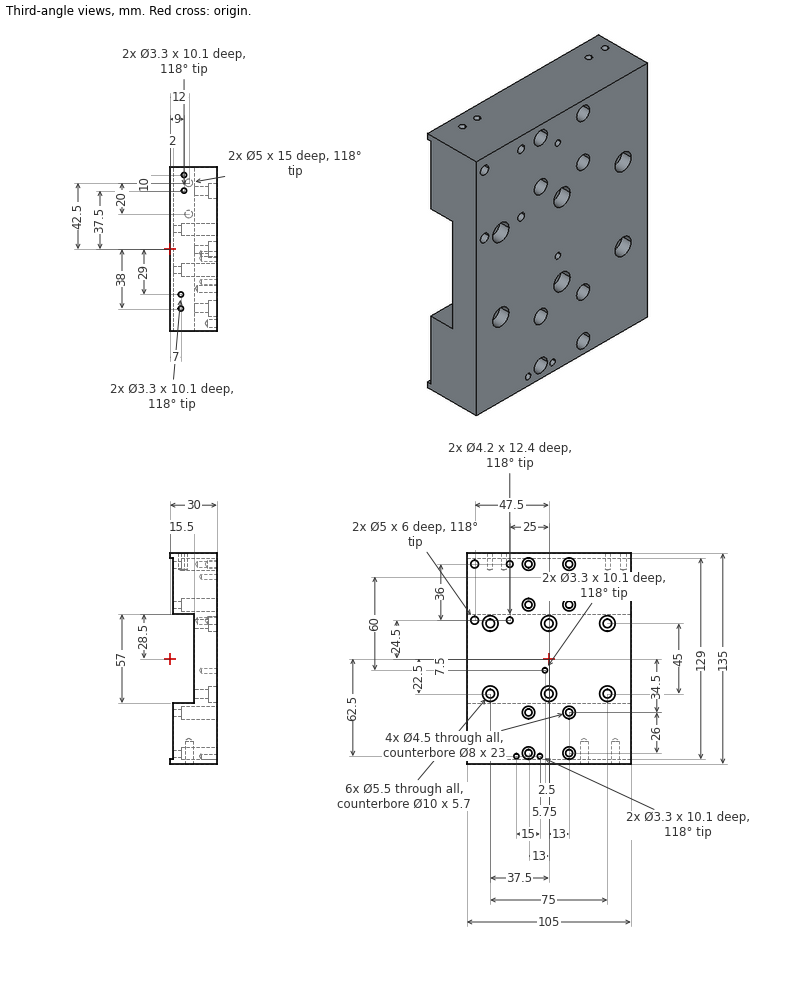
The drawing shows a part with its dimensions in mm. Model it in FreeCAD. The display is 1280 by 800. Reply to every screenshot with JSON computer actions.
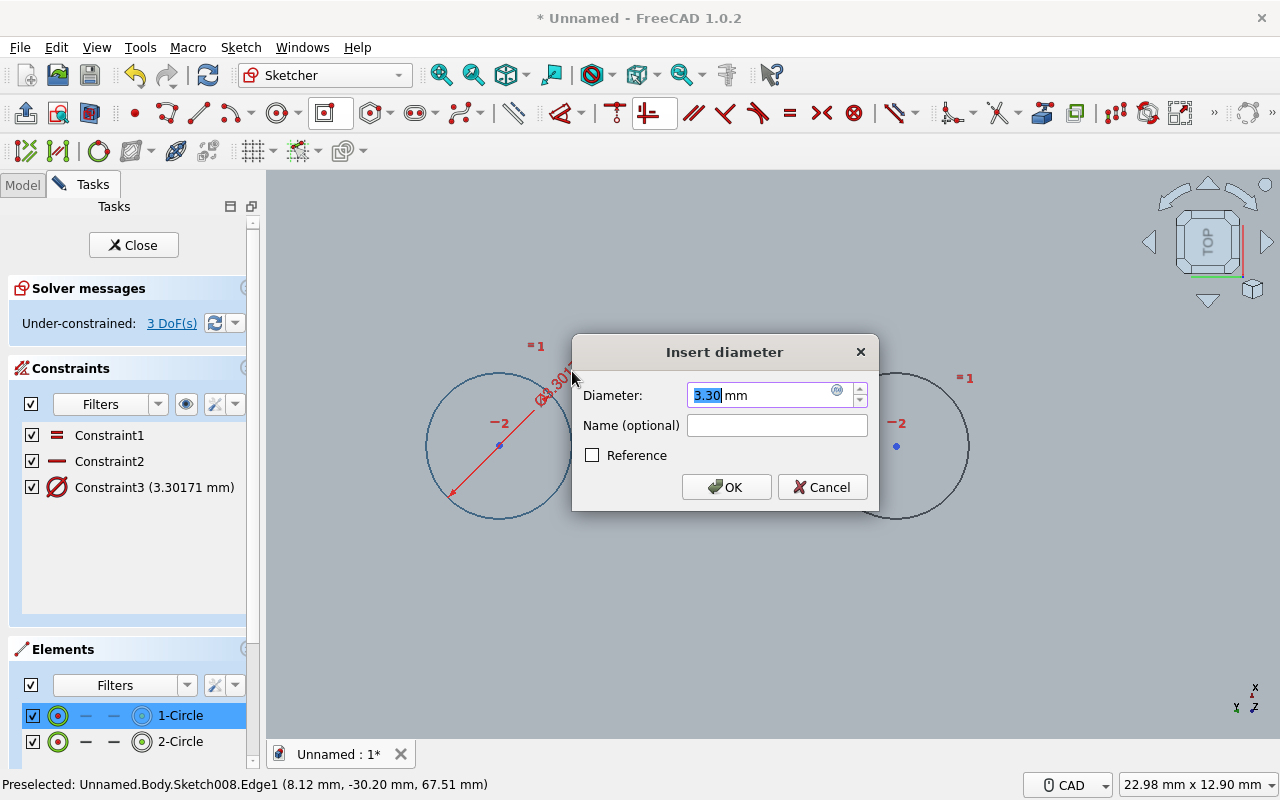
{"action": "type", "text": "3.3"}
{"action": "key", "text": "Return"}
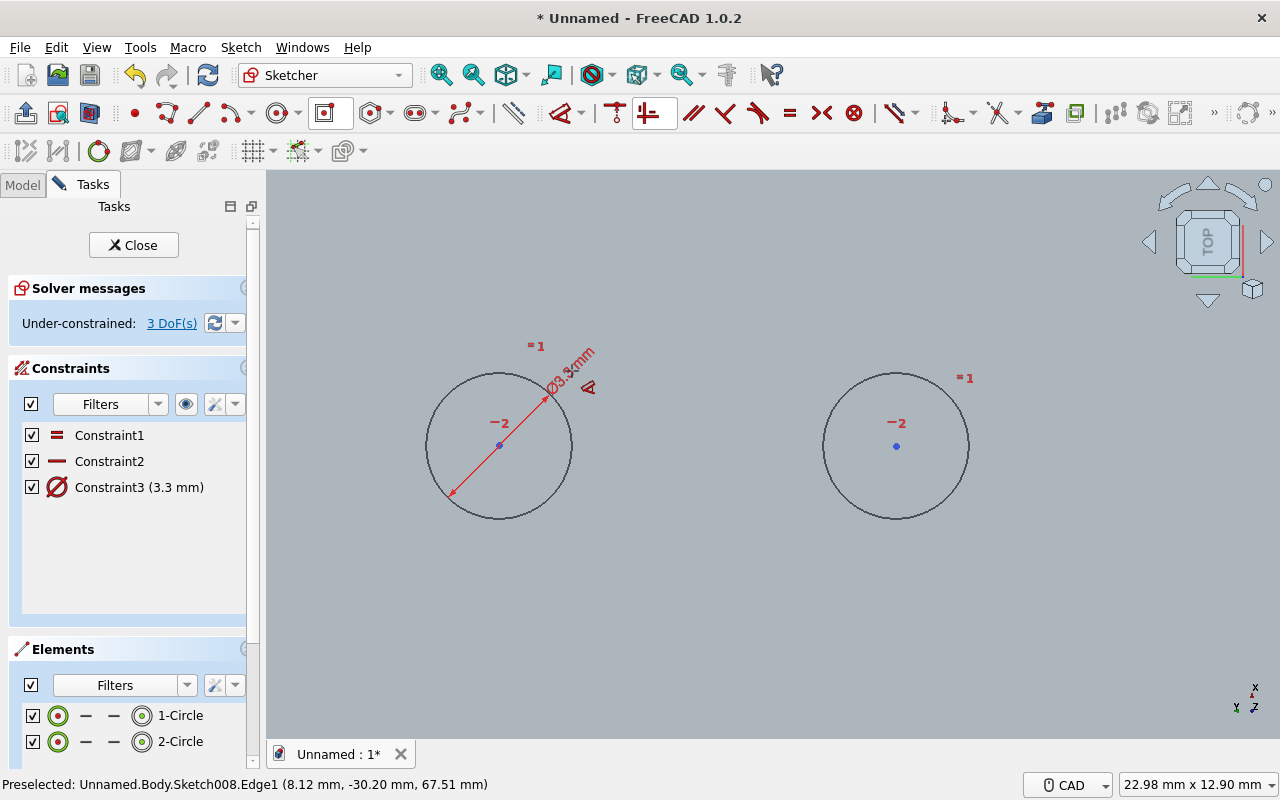
{"action": "left_click", "coordinate": [499, 446]}
{"action": "left_click", "coordinate": [533, 578]}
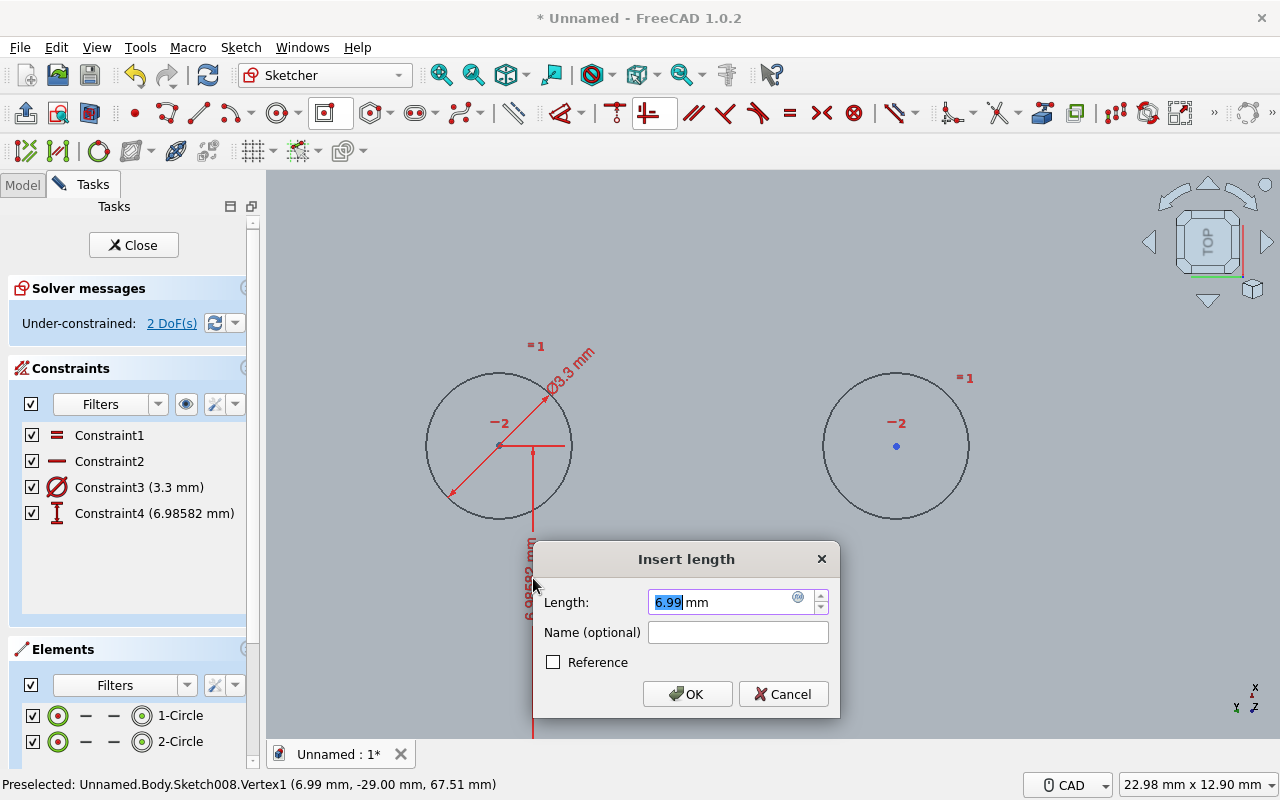
{"action": "type", "text": "7"}
{"action": "key", "text": "Return"}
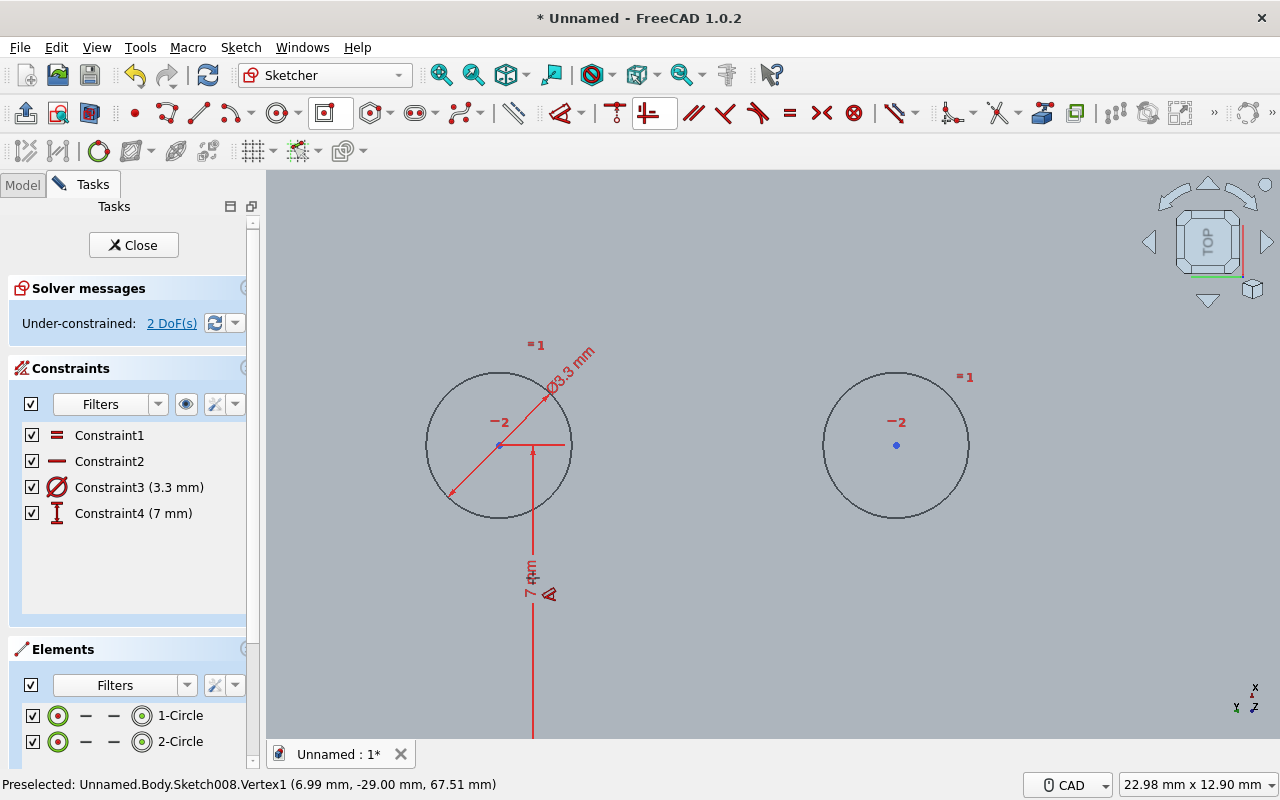
{"action": "left_click", "coordinate": [499, 445]}
{"action": "left_click", "coordinate": [396, 411]}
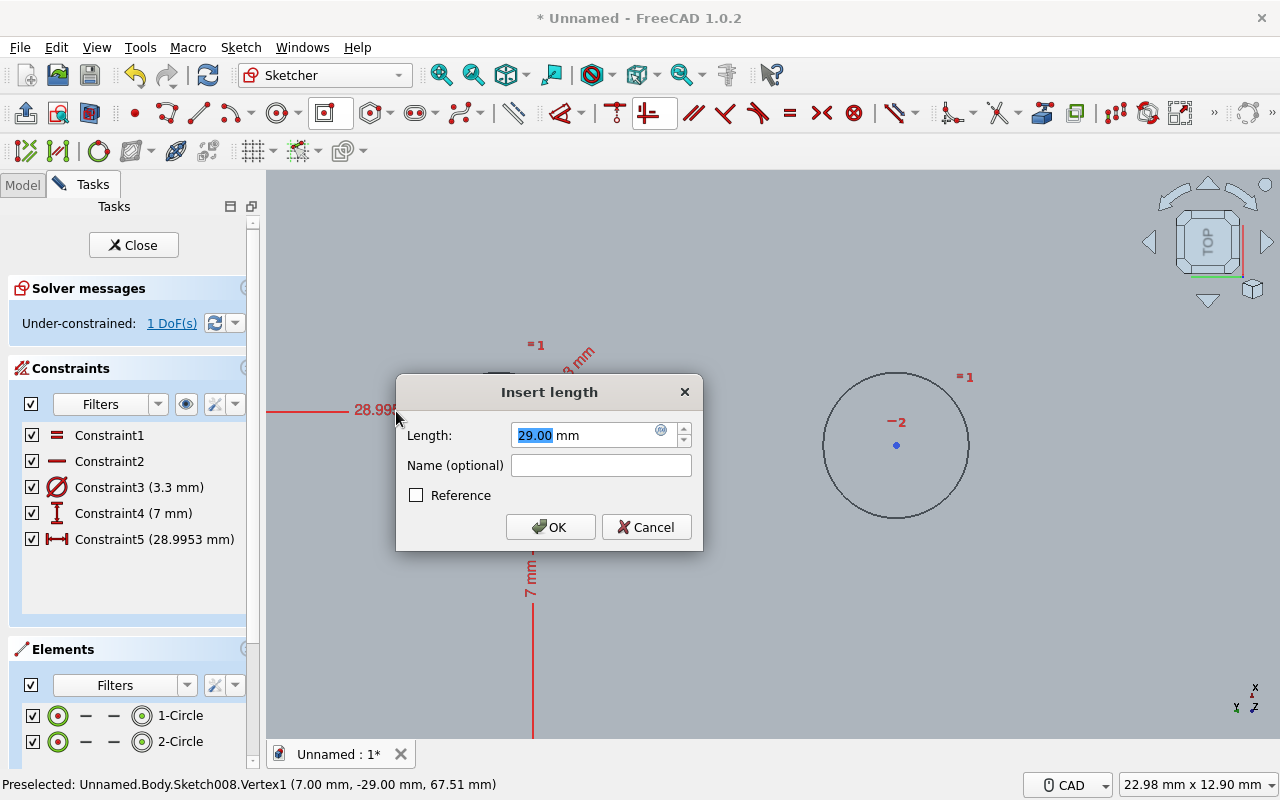
{"action": "type", "text": "29"}
{"action": "key", "text": "Return"}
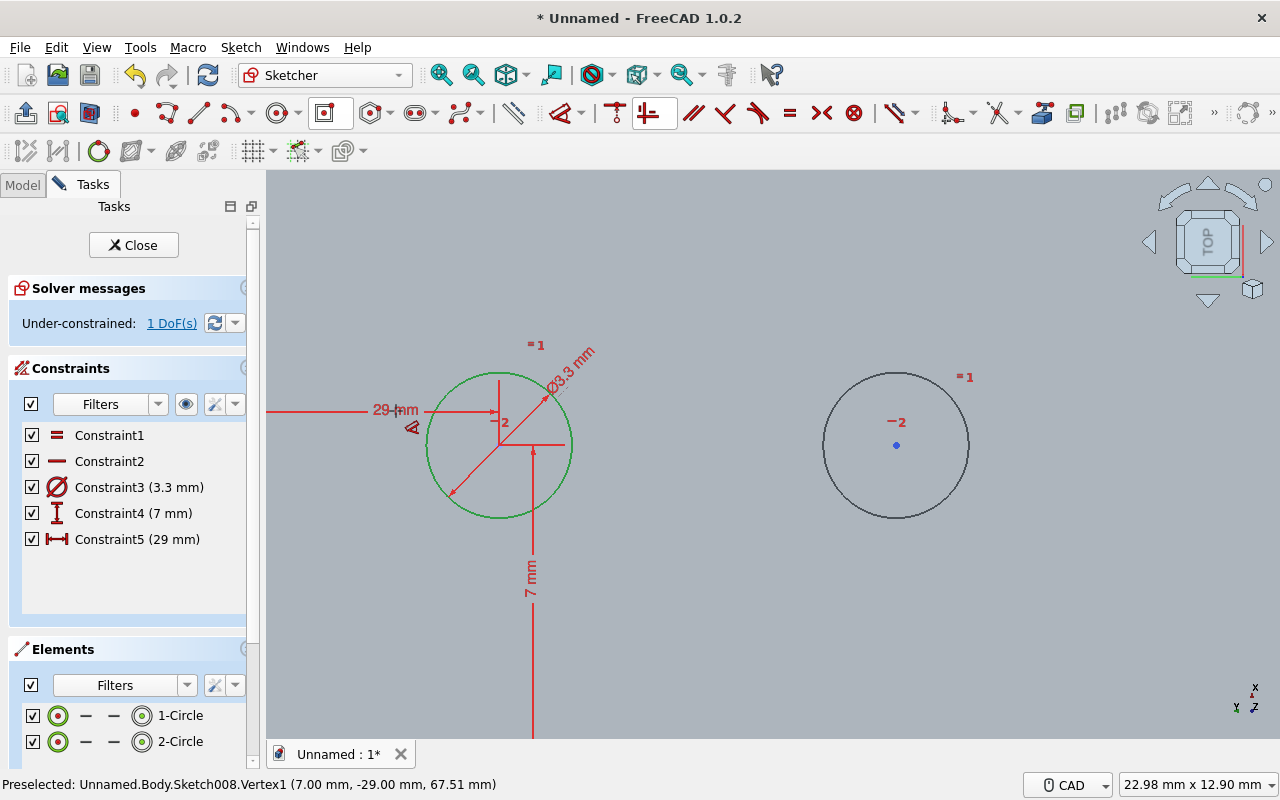
{"action": "left_click", "coordinate": [896, 445]}
{"action": "left_click", "coordinate": [595, 411]}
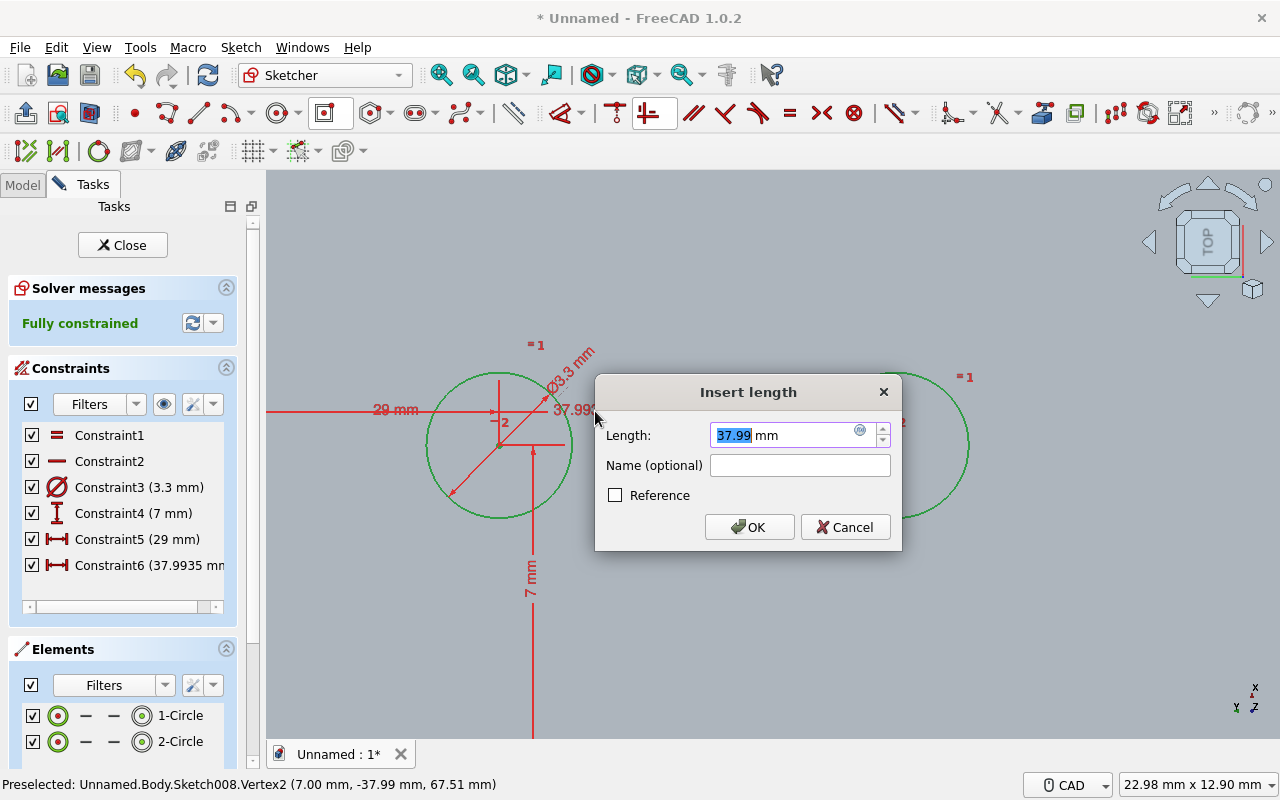
{"action": "type", "text": "38"}
{"action": "key", "text": "Return"}
{"action": "key", "text": "Escape"}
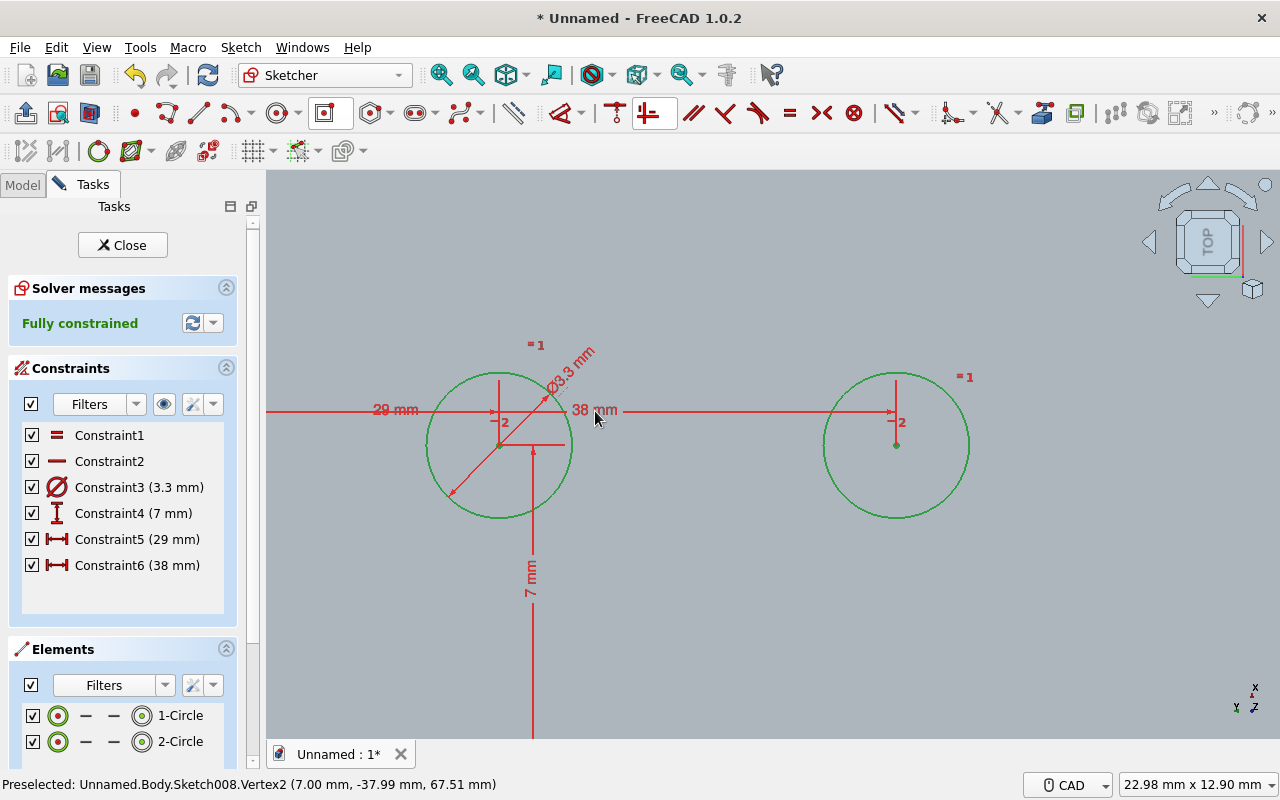
{"action": "left_click", "coordinate": [123, 245]}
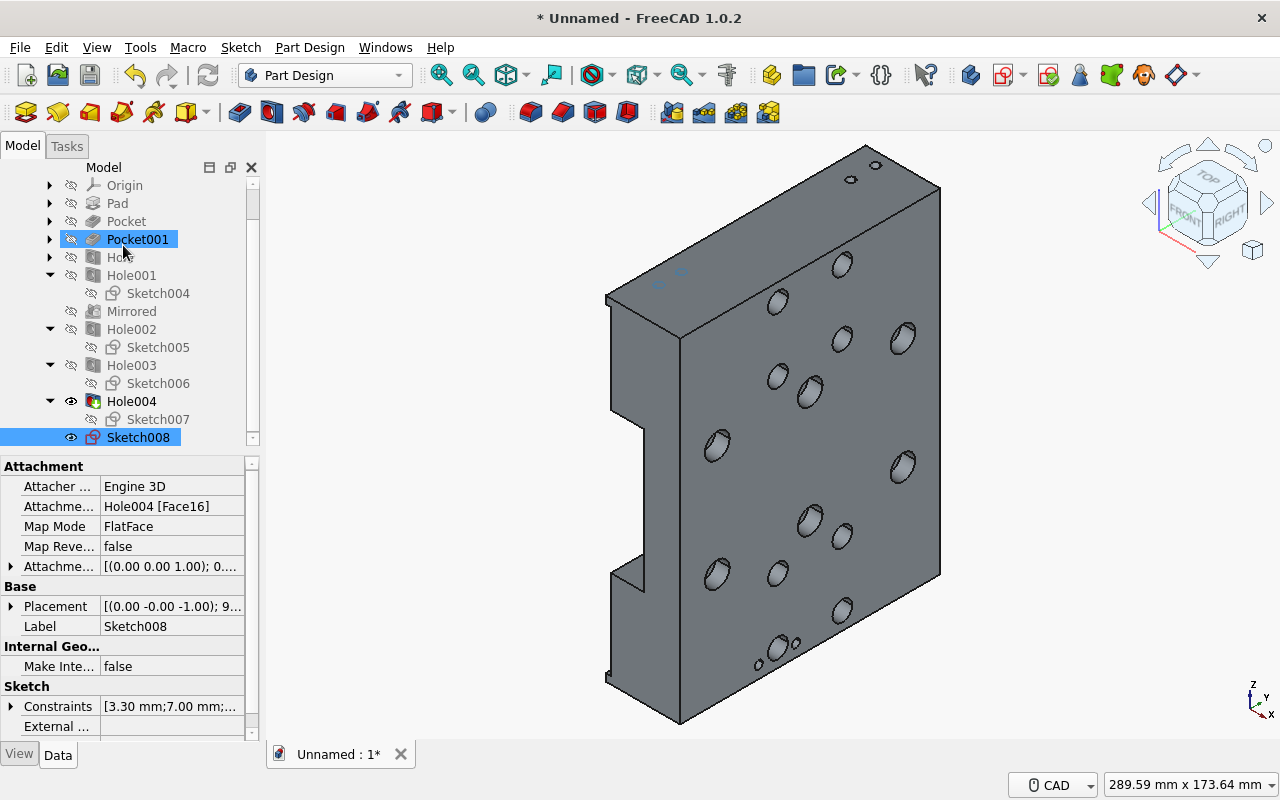
{"action": "left_click", "coordinate": [272, 112]}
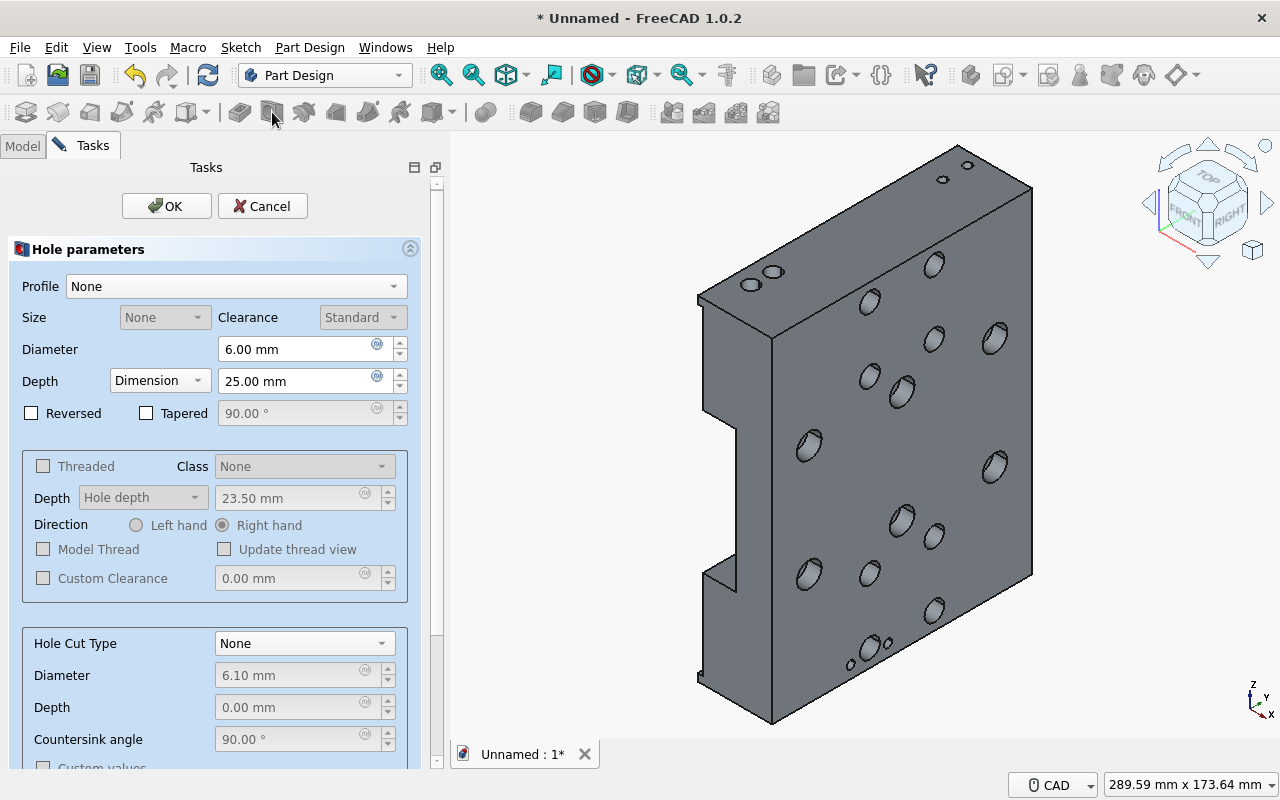
{"action": "triple_click", "coordinate": [305, 349]}